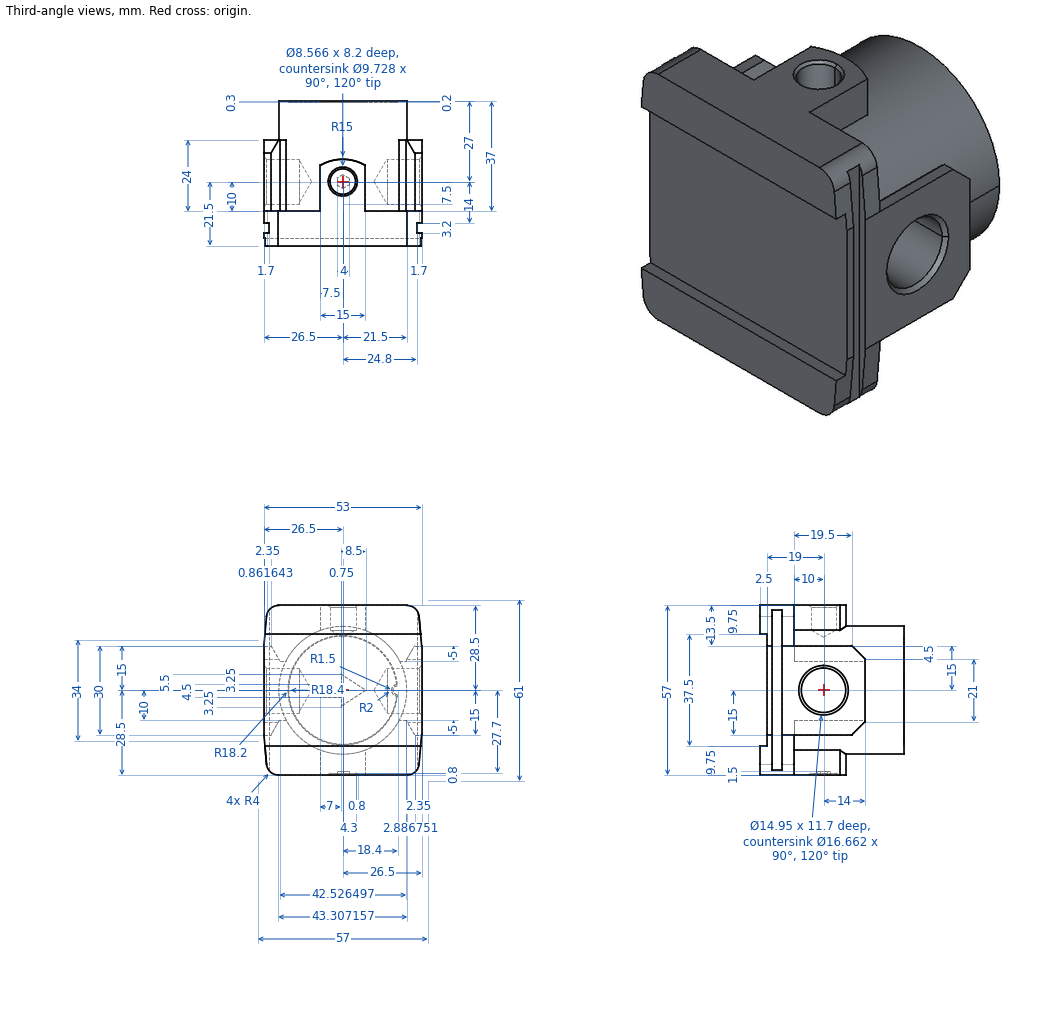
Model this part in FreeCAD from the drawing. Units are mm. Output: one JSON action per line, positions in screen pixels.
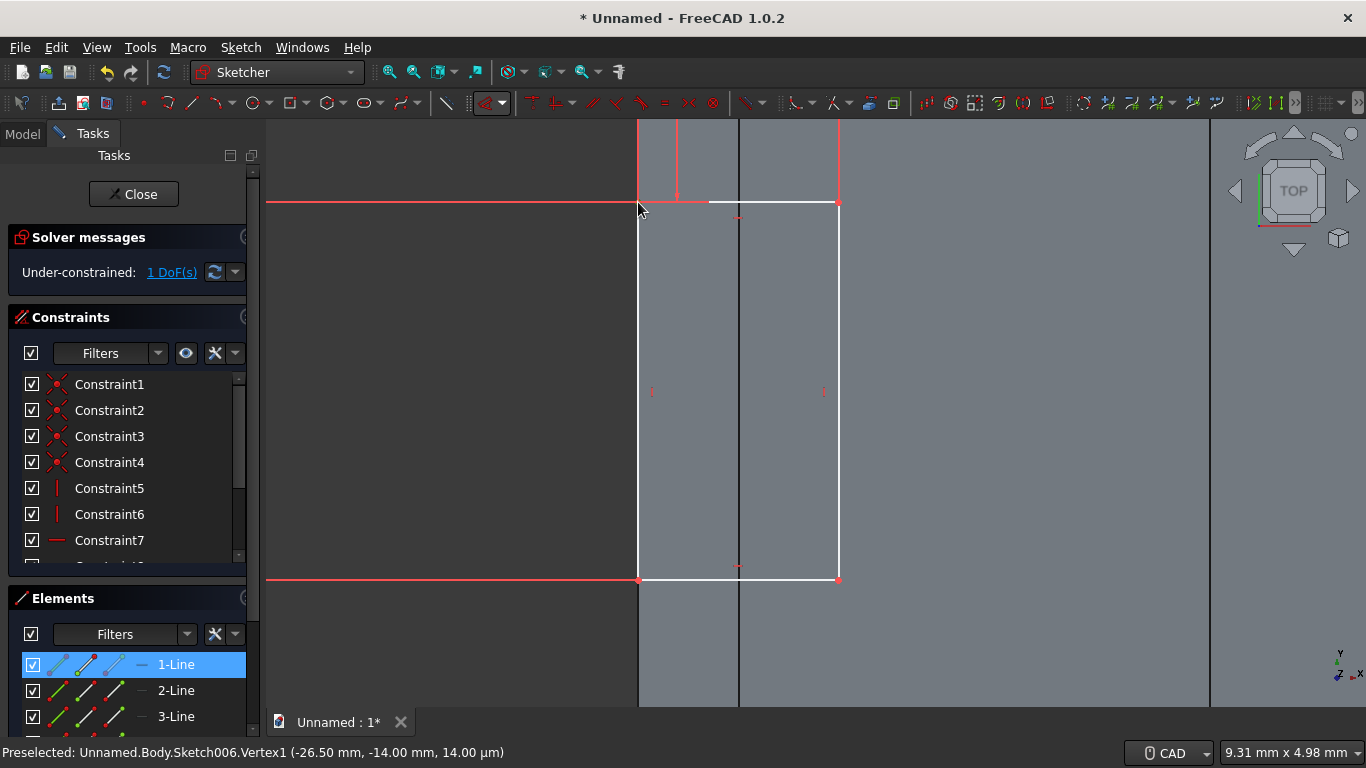
{"action": "key", "text": "l"}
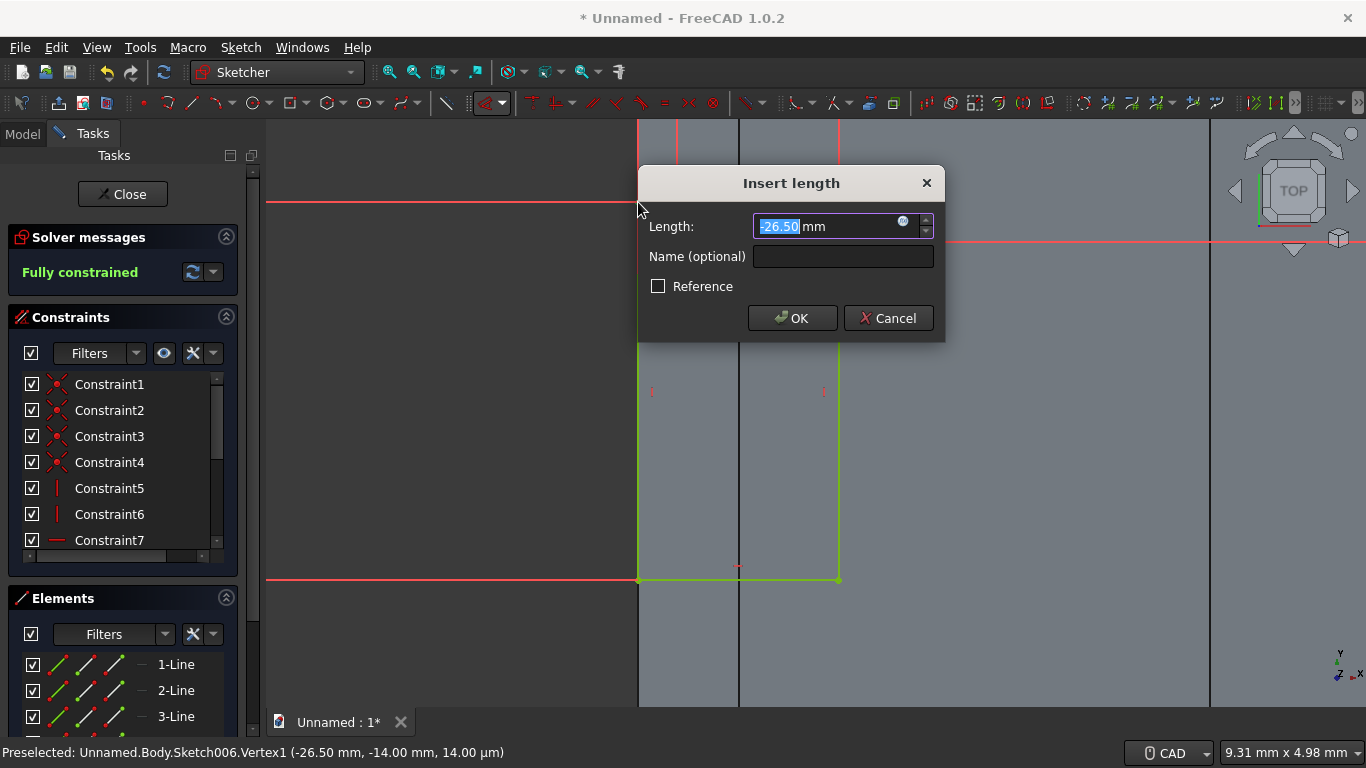
{"action": "type", "text": "-26.5"}
{"action": "key", "text": "Return"}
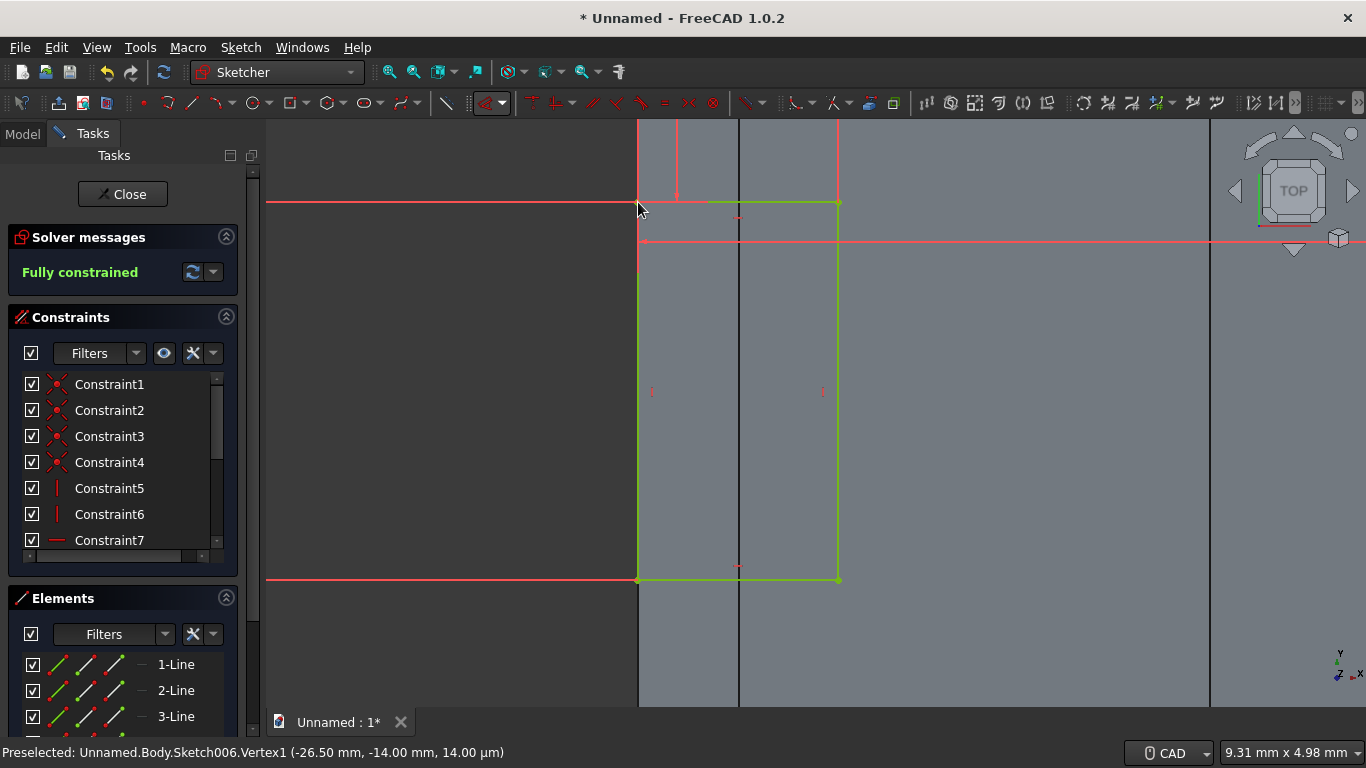
{"action": "left_click", "coordinate": [123, 194]}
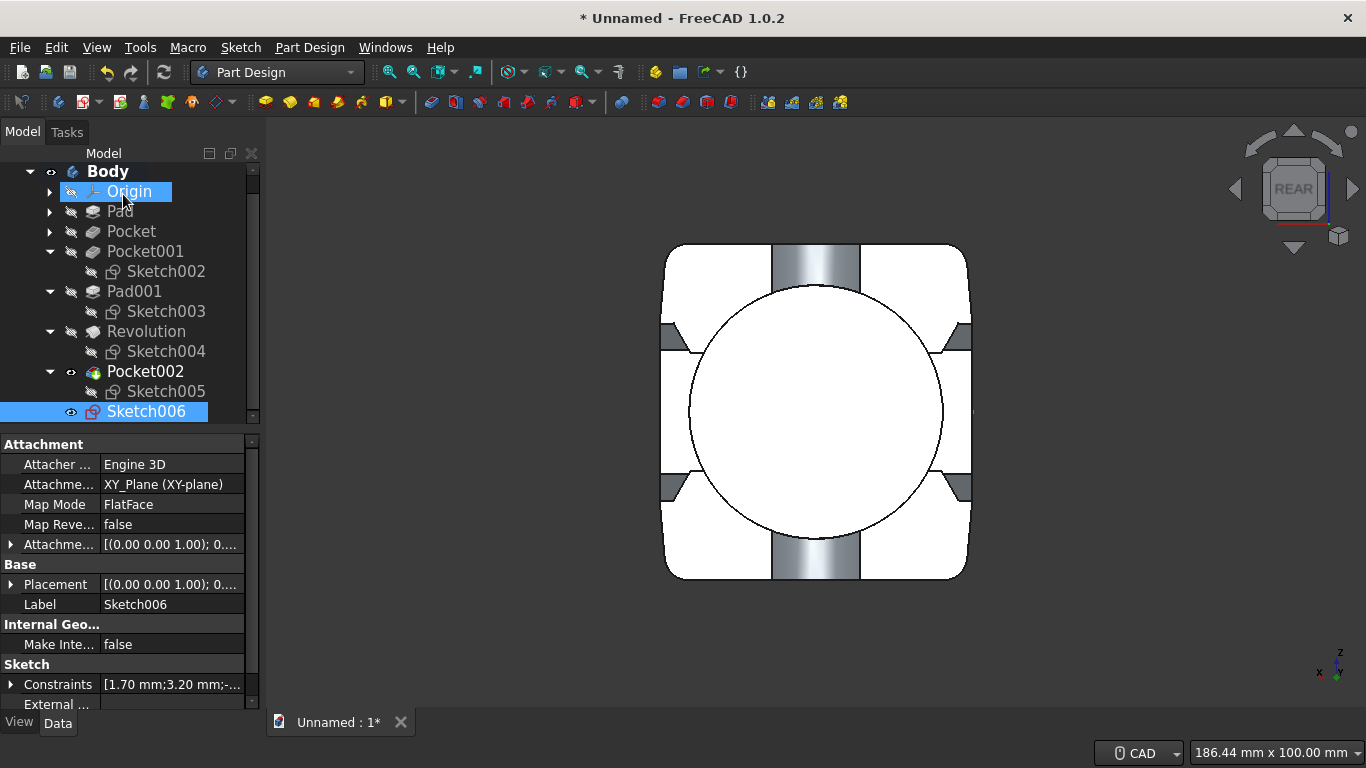
{"action": "left_click", "coordinate": [432, 102]}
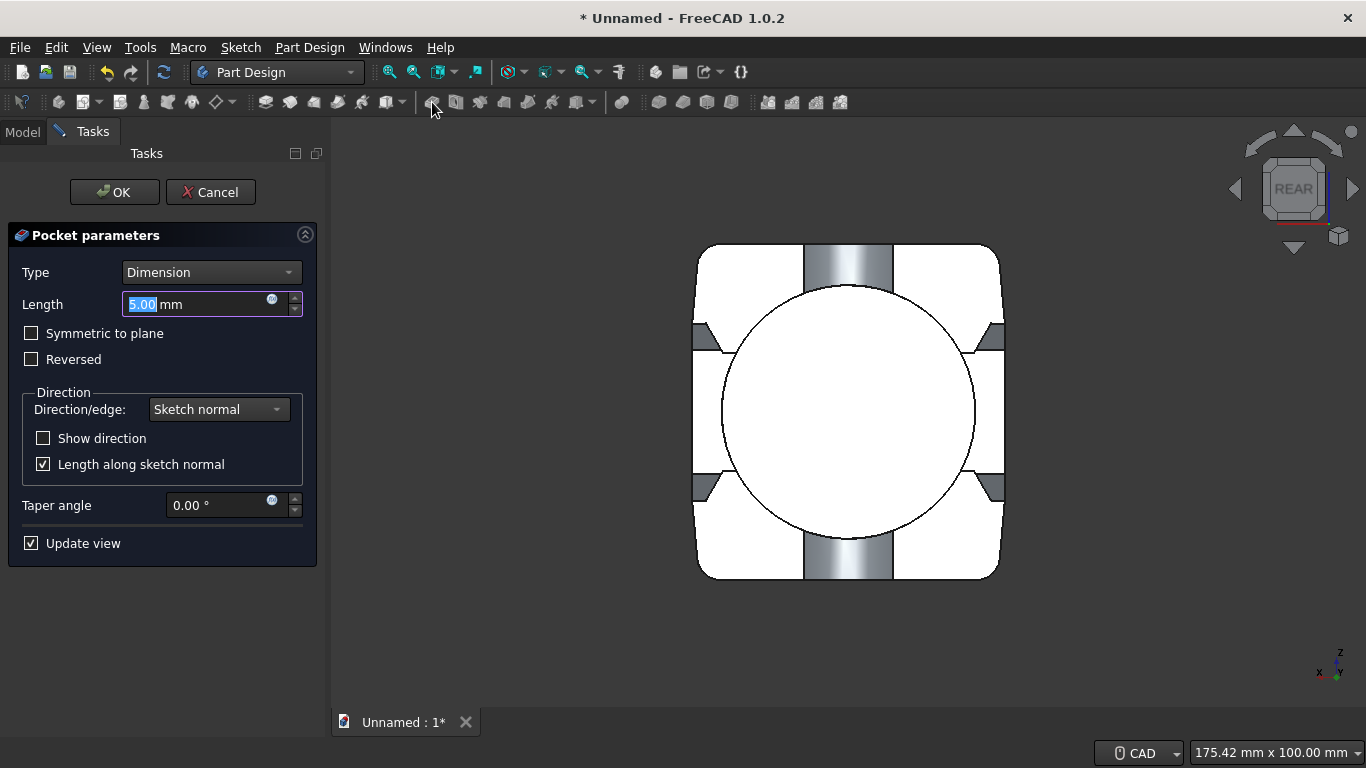
{"action": "type", "text": "57"}
{"action": "key", "text": "Tab"}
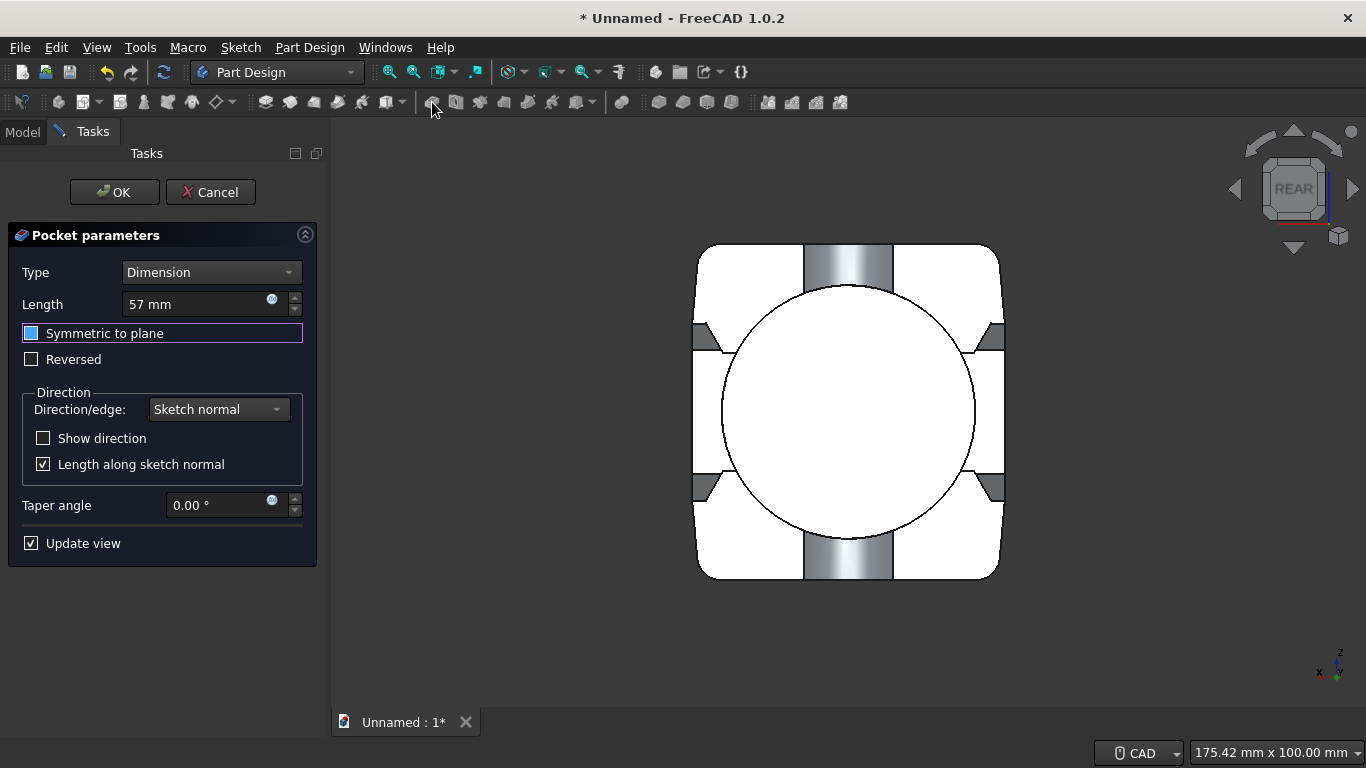
{"action": "left_click", "coordinate": [30, 333]}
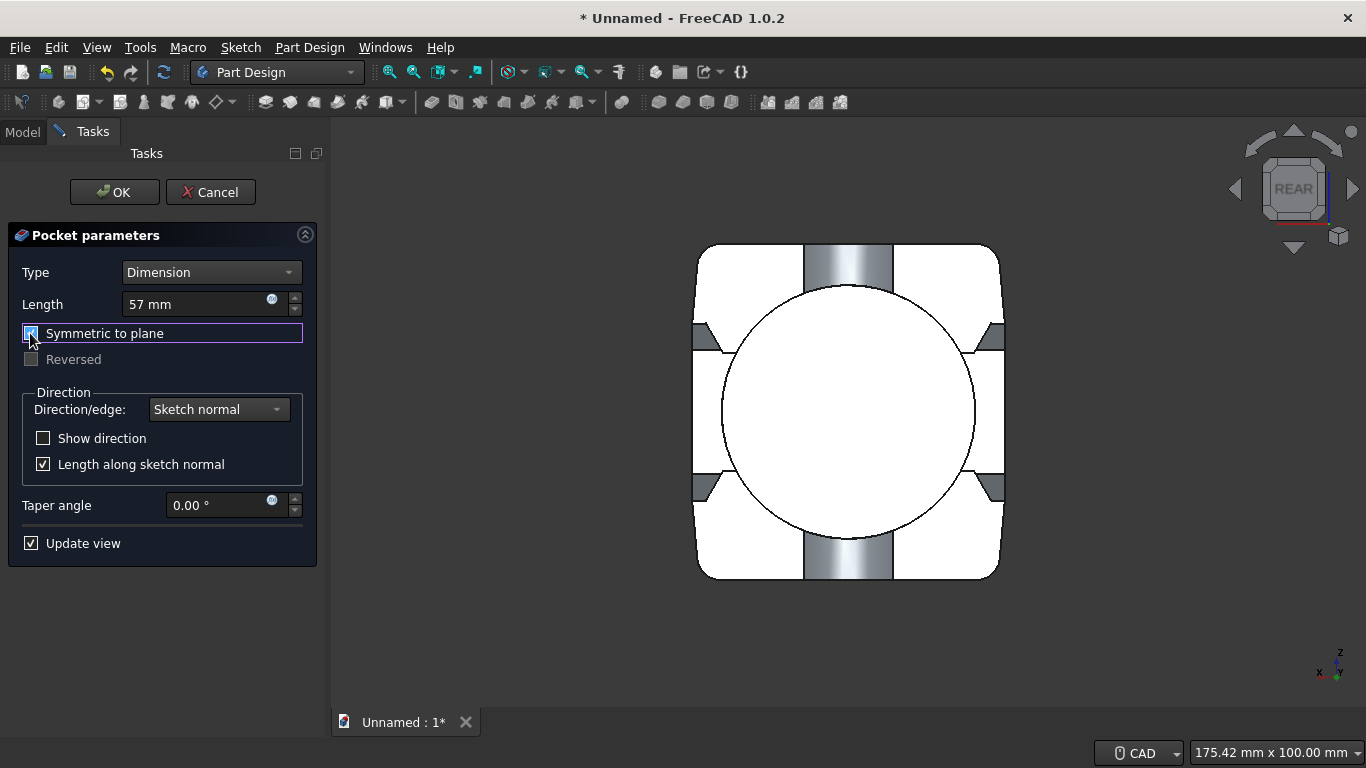
{"action": "left_click", "coordinate": [115, 192]}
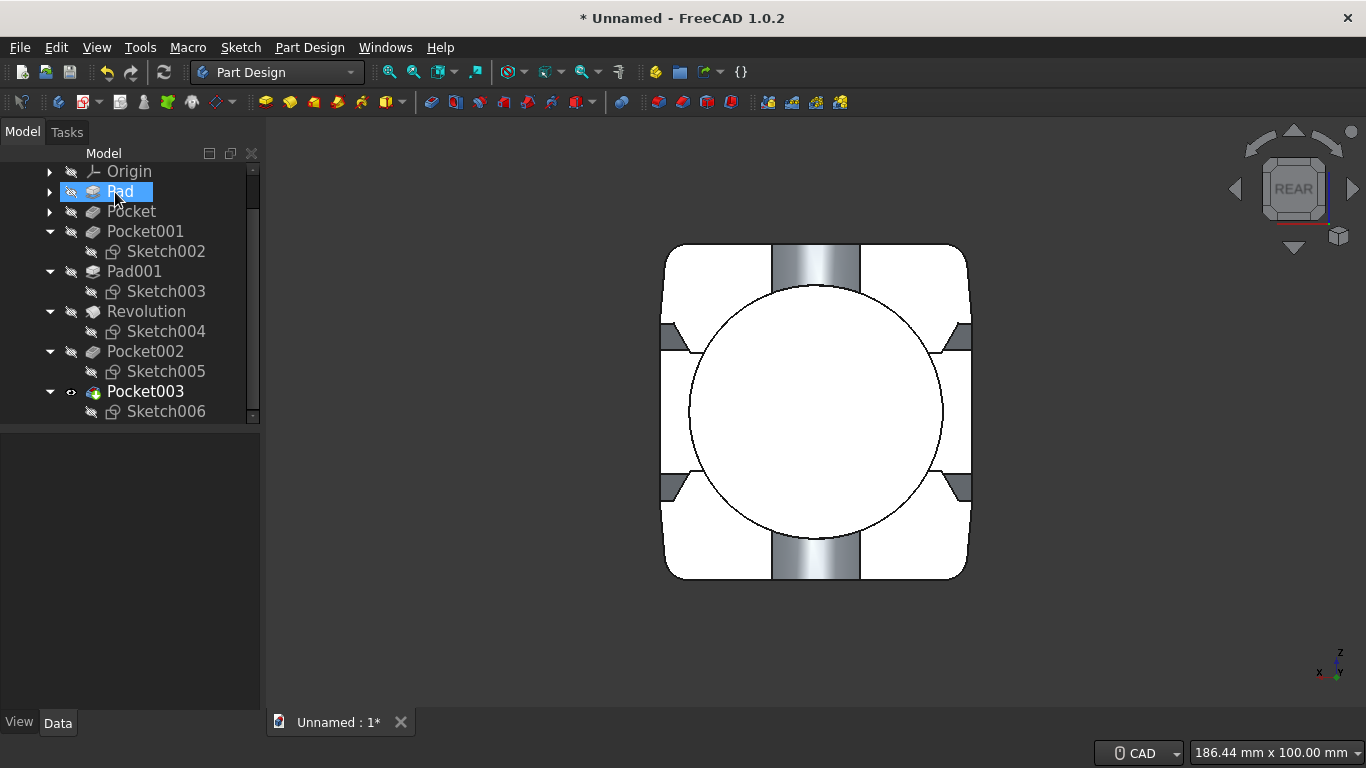
{"action": "left_click", "coordinate": [84, 102]}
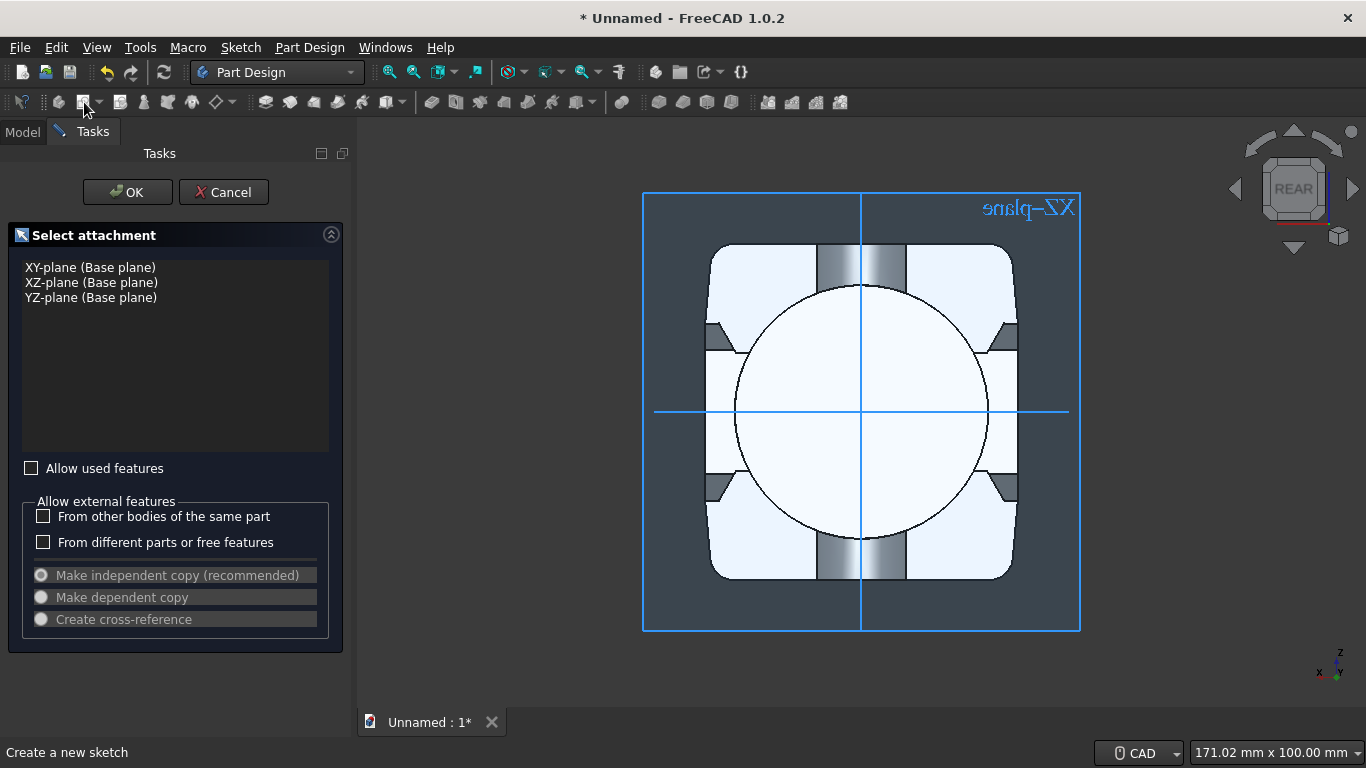
{"action": "left_click", "coordinate": [82, 282]}